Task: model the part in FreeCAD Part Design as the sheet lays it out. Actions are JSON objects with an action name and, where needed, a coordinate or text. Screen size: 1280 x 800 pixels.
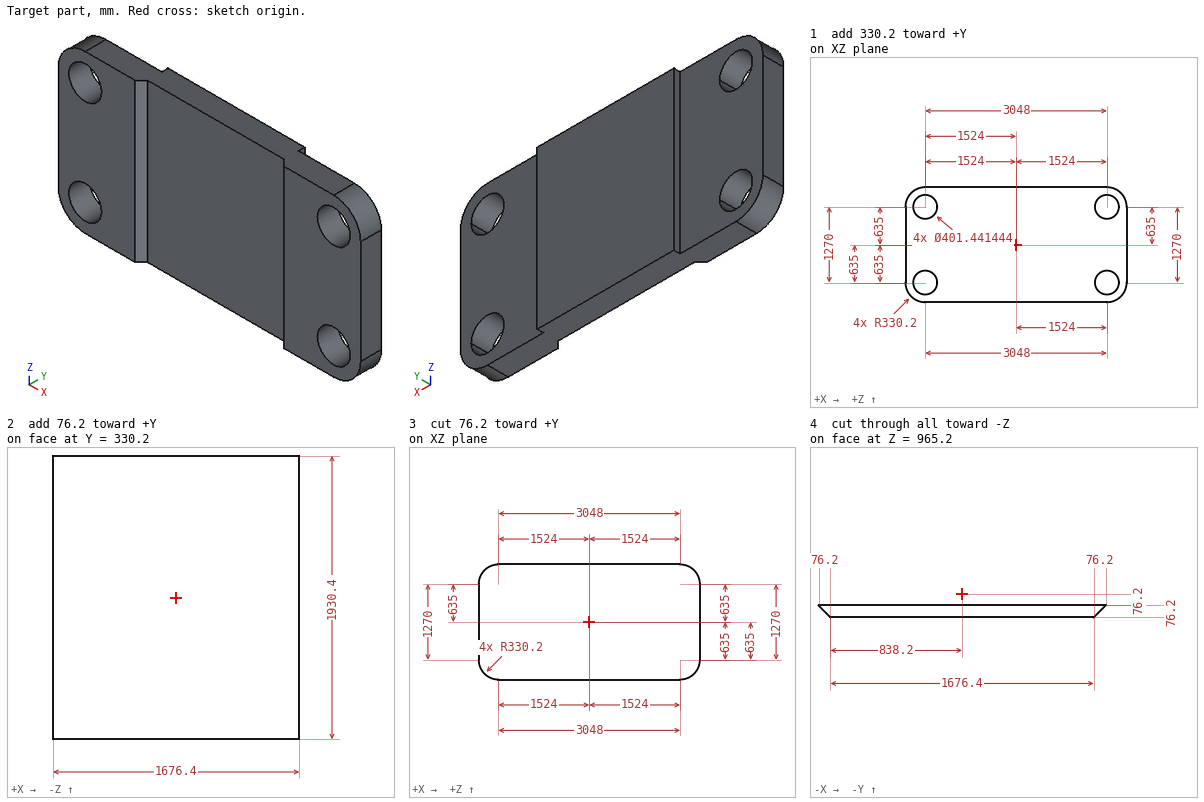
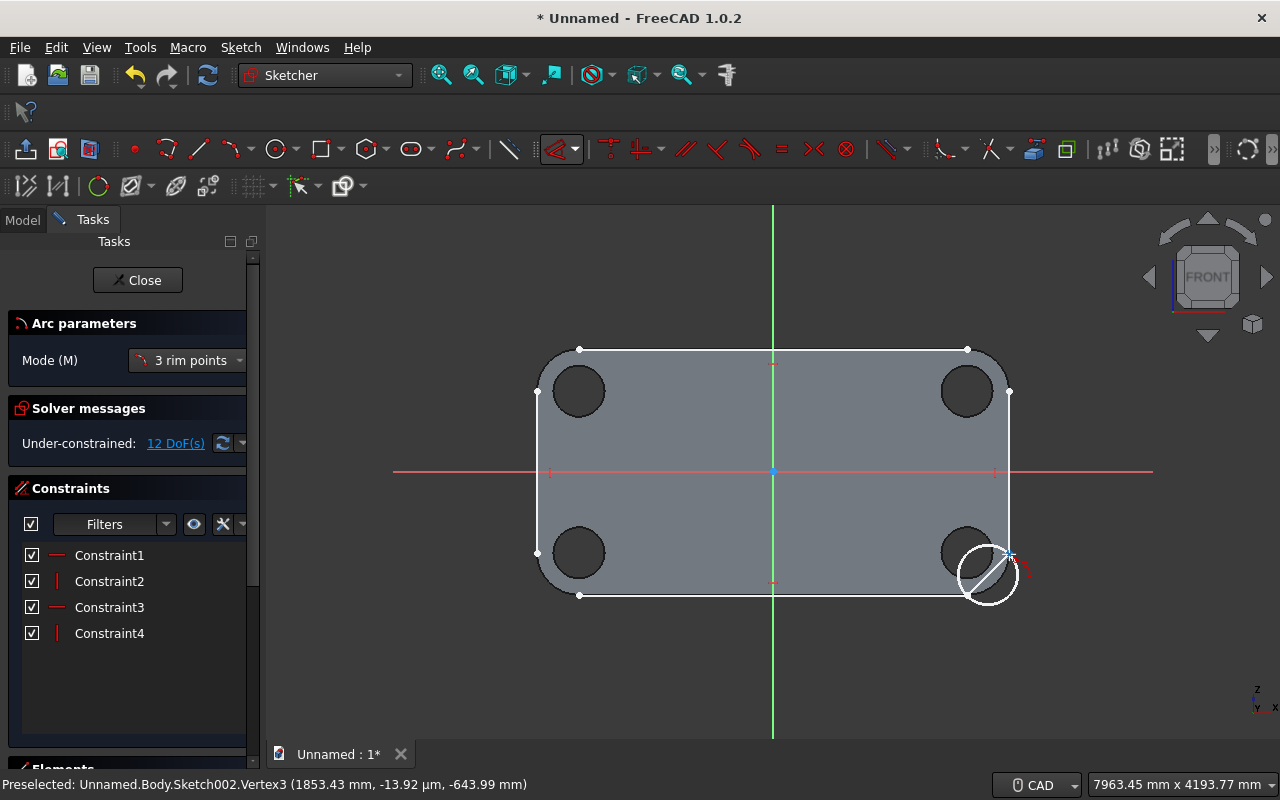
{"action": "scroll", "coordinate": [997, 583], "scroll_direction": "up", "scroll_amount": 2}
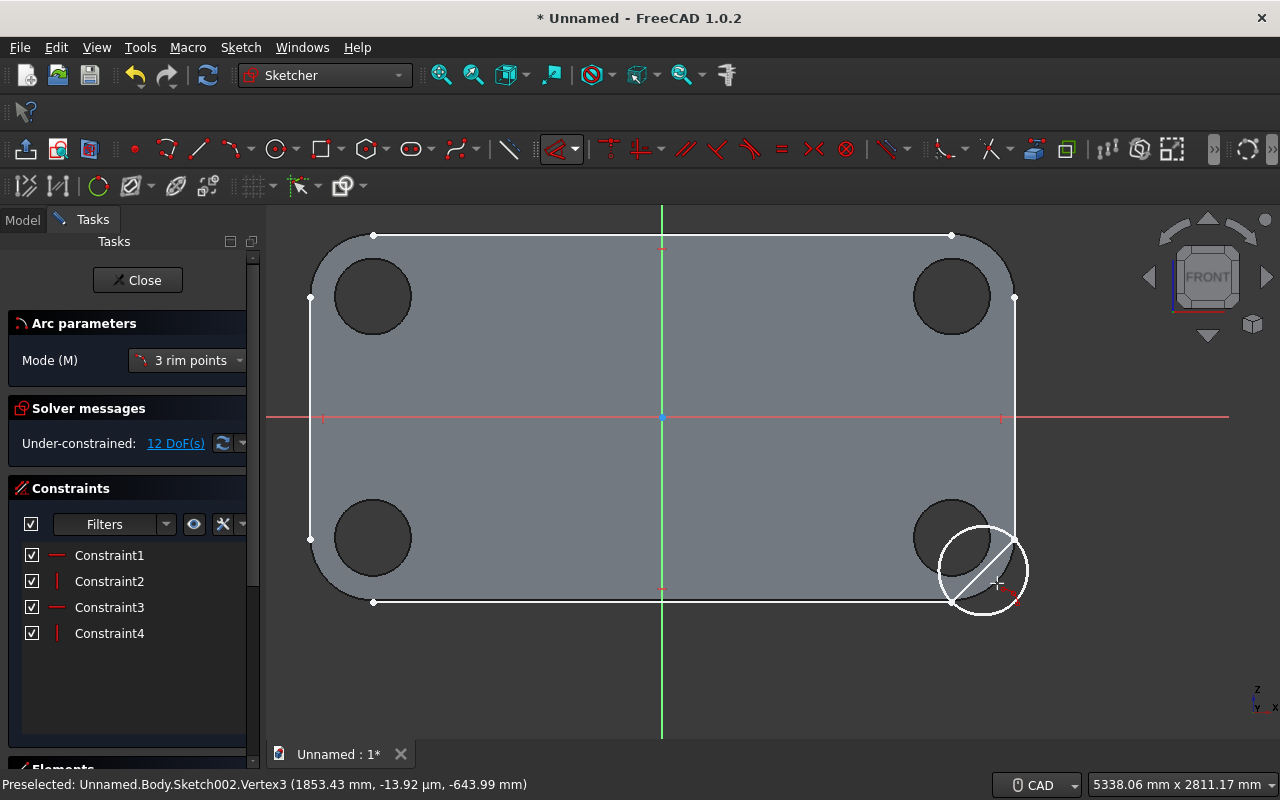
{"action": "left_click", "coordinate": [996, 582]}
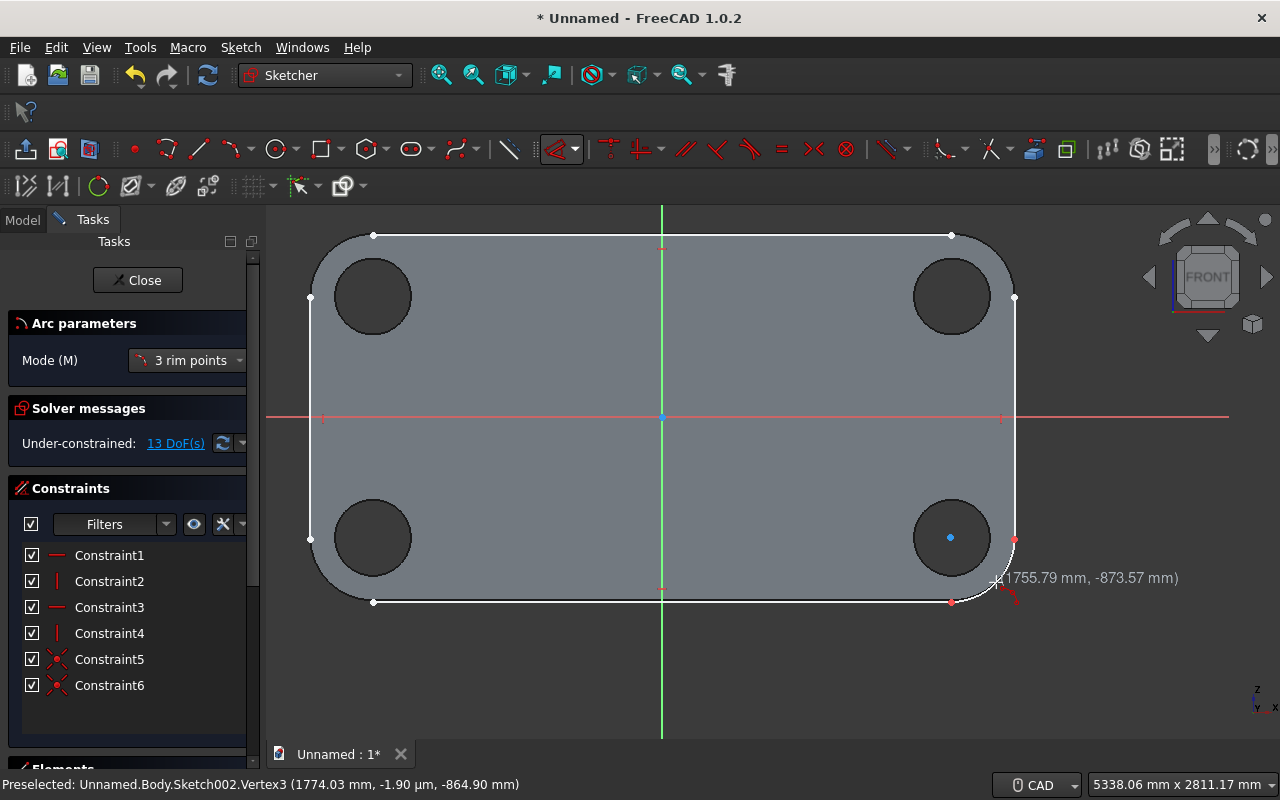
{"action": "left_click", "coordinate": [1015, 298]}
{"action": "left_click", "coordinate": [952, 235]}
{"action": "left_click", "coordinate": [996, 252]}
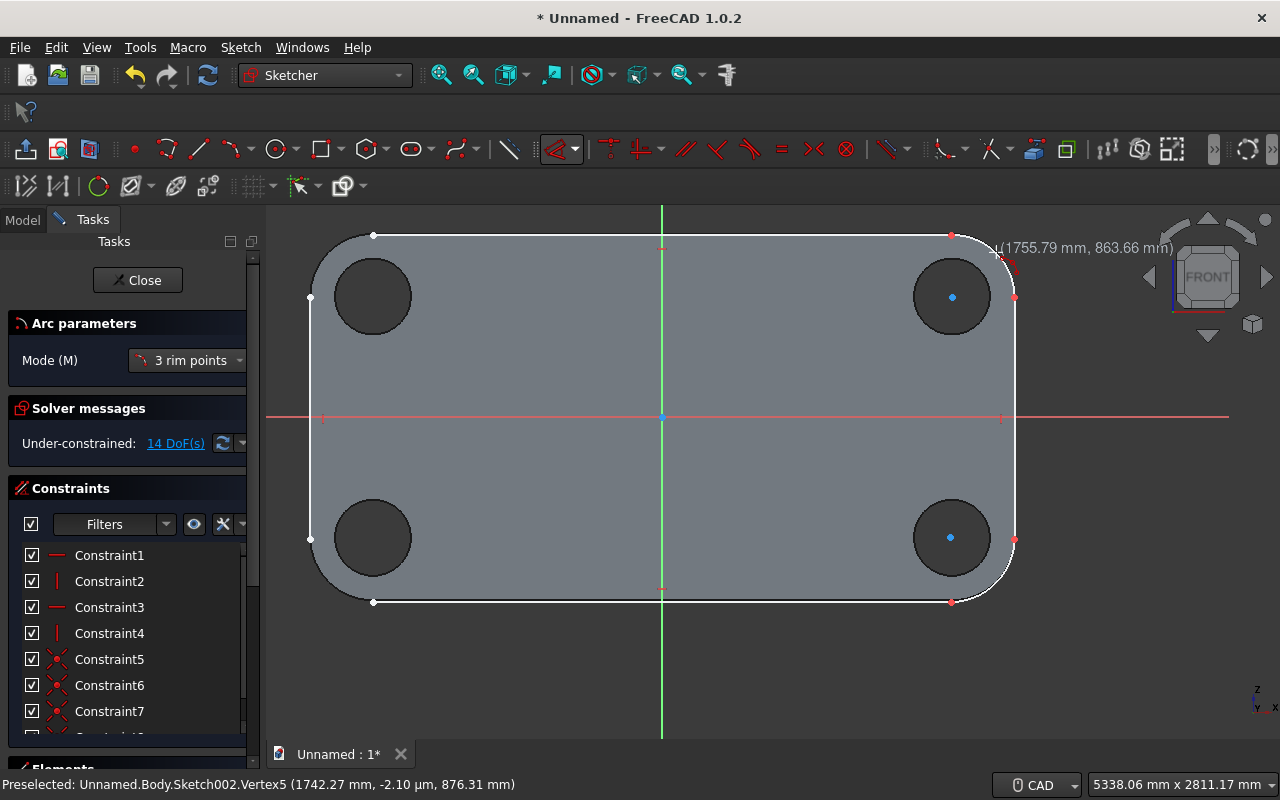
{"action": "left_click", "coordinate": [373, 235]}
{"action": "left_click", "coordinate": [310, 298]}
{"action": "left_click", "coordinate": [329, 252]}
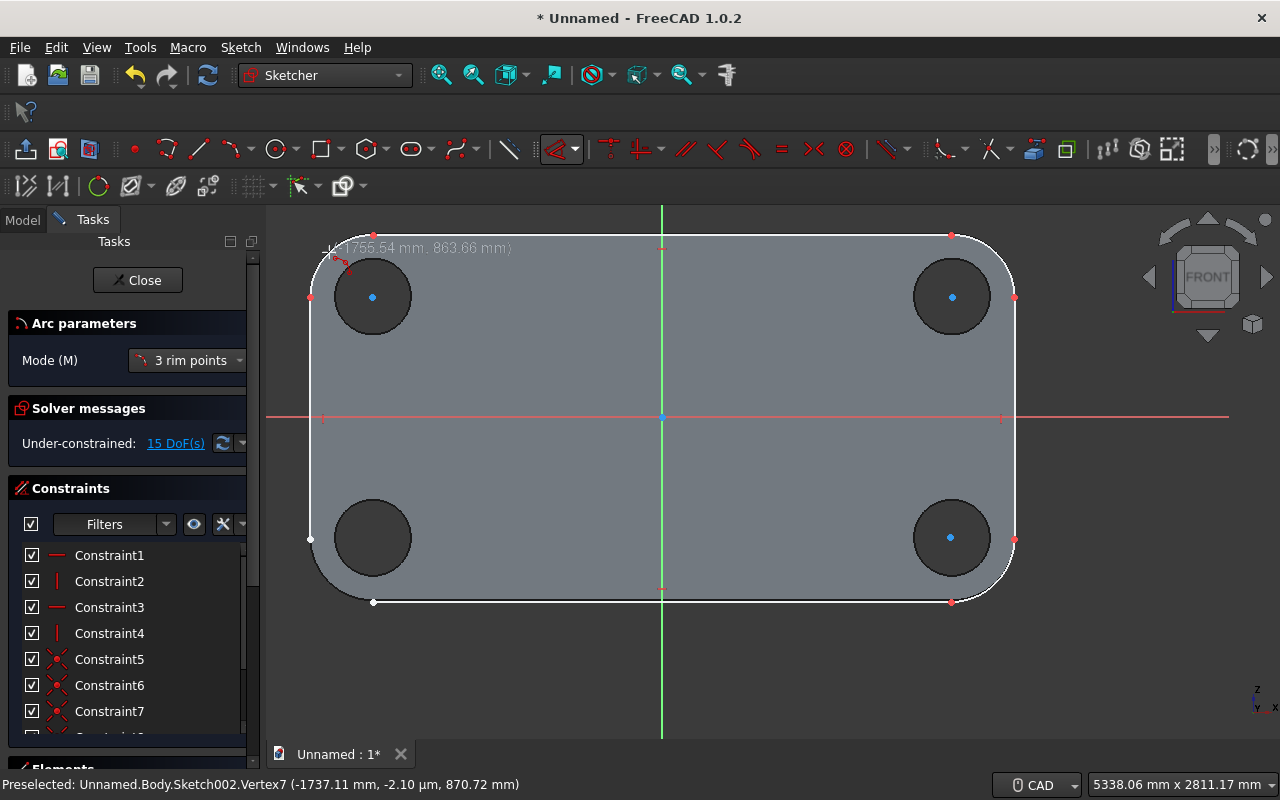
{"action": "left_click", "coordinate": [310, 539]}
{"action": "left_click", "coordinate": [373, 602]}
{"action": "left_click", "coordinate": [329, 582]}
{"action": "key", "text": "Escape"}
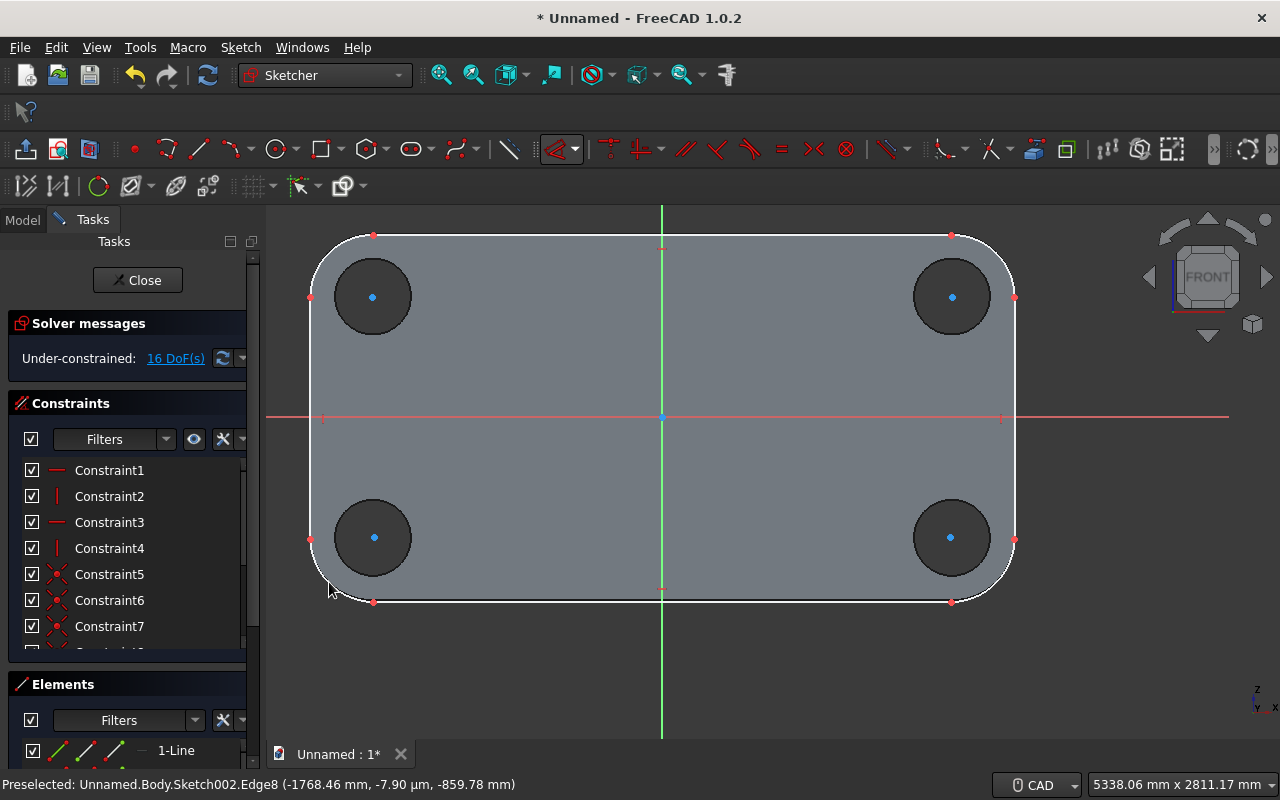
{"action": "left_click", "coordinate": [980, 595]}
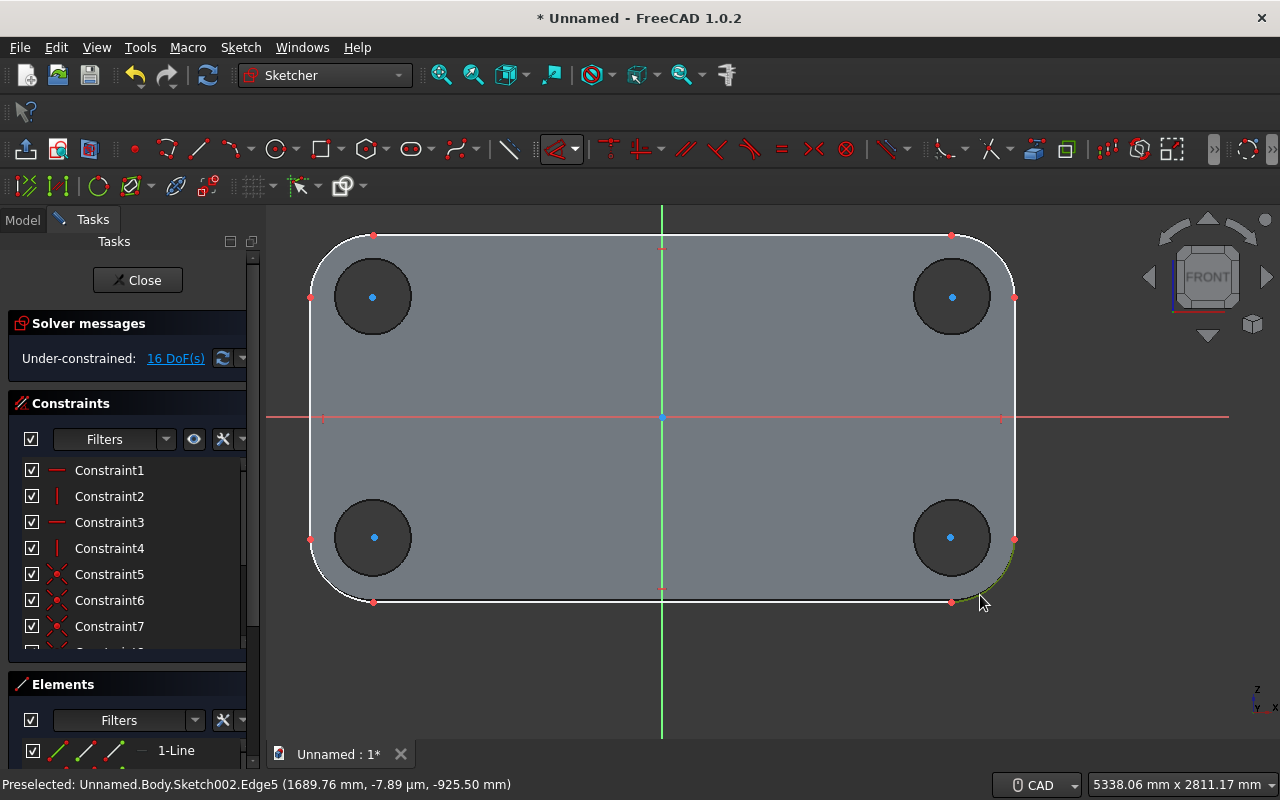
{"action": "left_click", "coordinate": [1008, 269]}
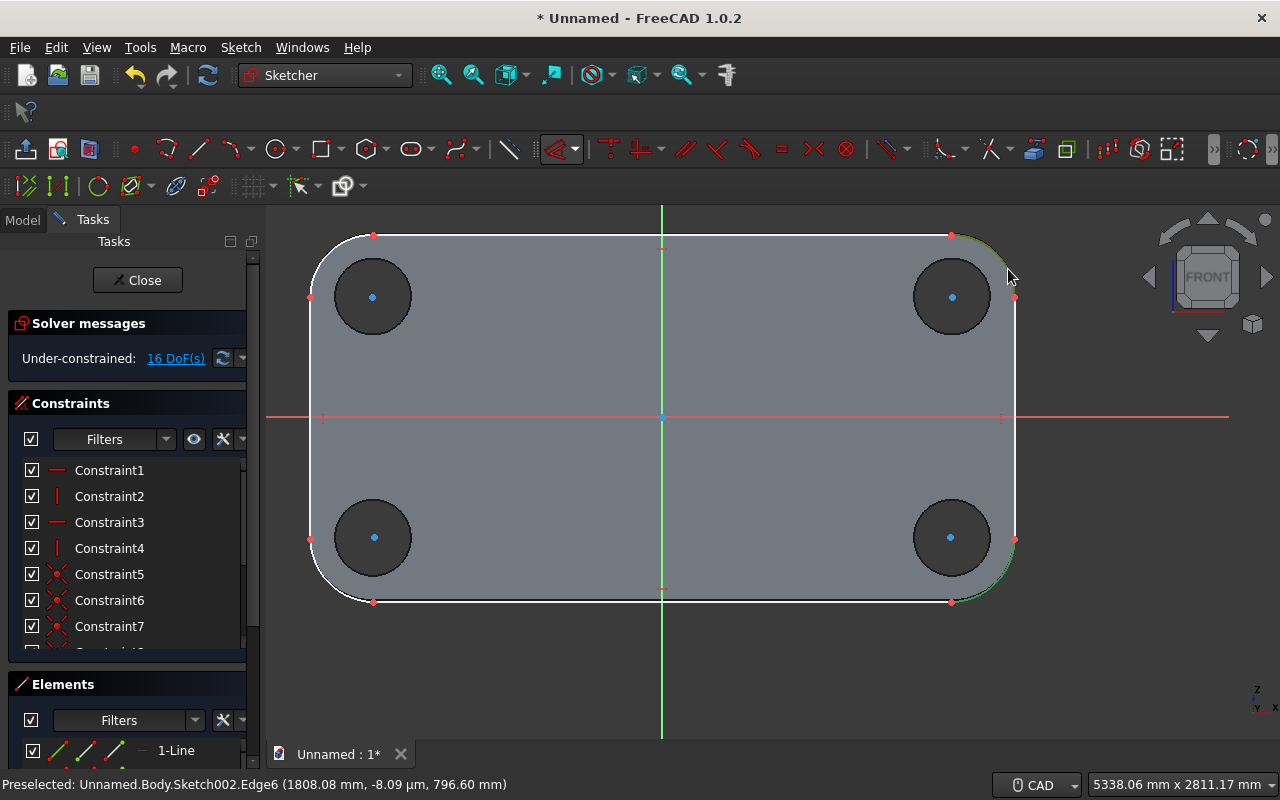
{"action": "left_click", "coordinate": [345, 242]}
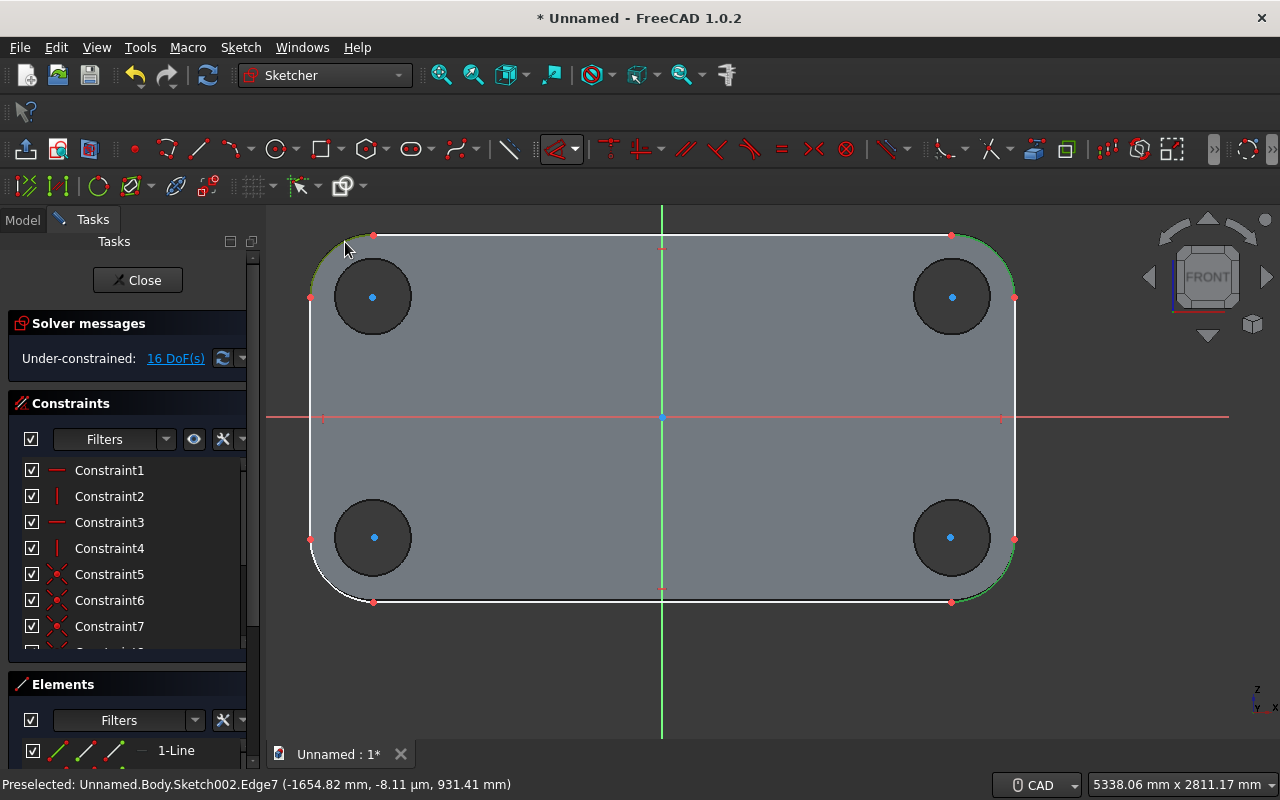
{"action": "left_click", "coordinate": [318, 568]}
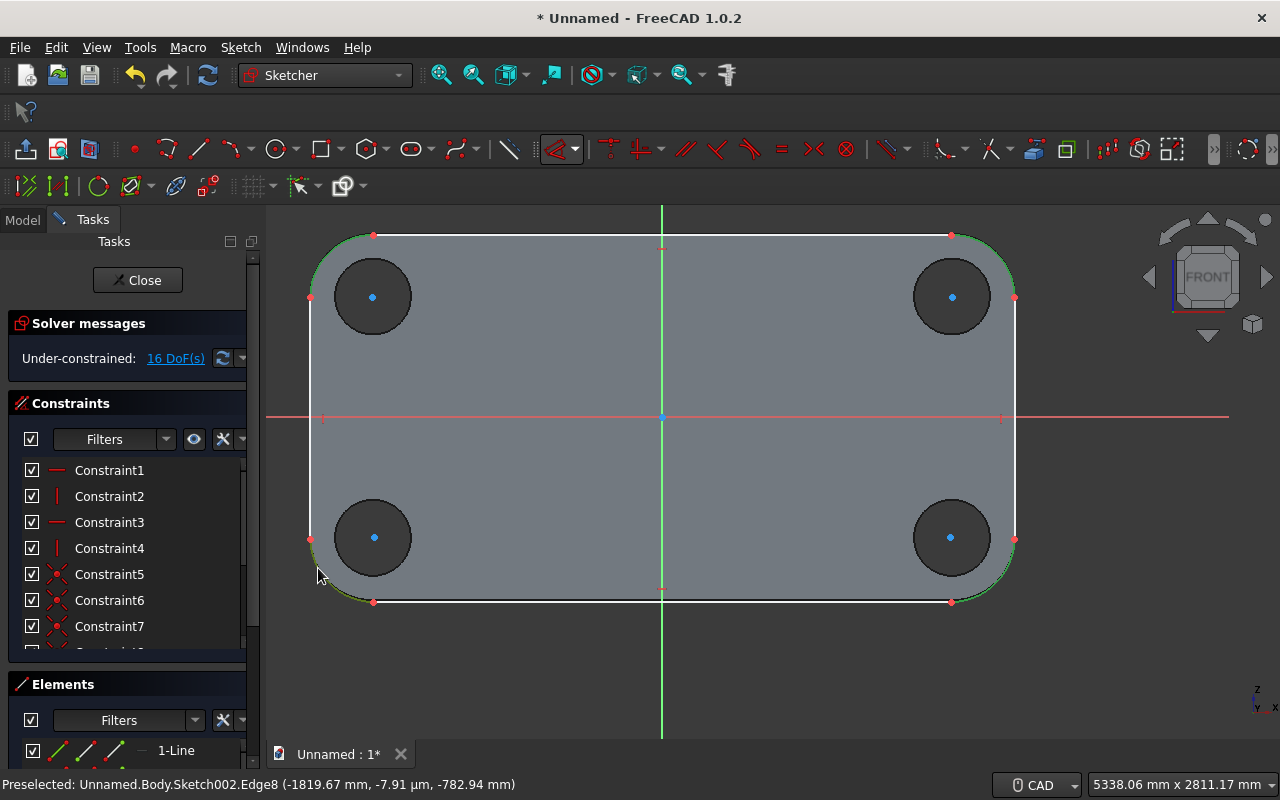
{"action": "left_click", "coordinate": [782, 150]}